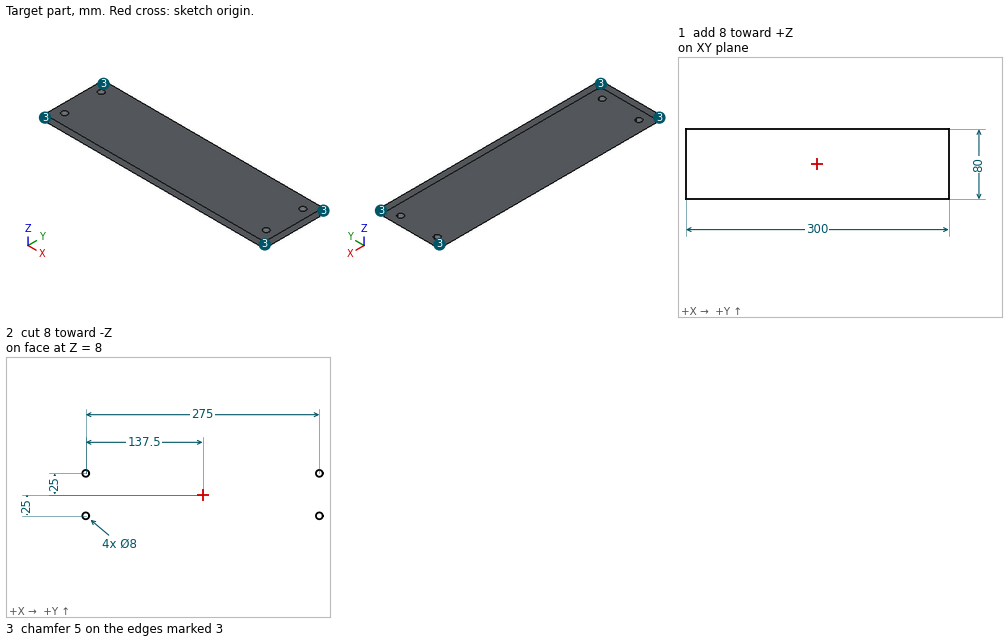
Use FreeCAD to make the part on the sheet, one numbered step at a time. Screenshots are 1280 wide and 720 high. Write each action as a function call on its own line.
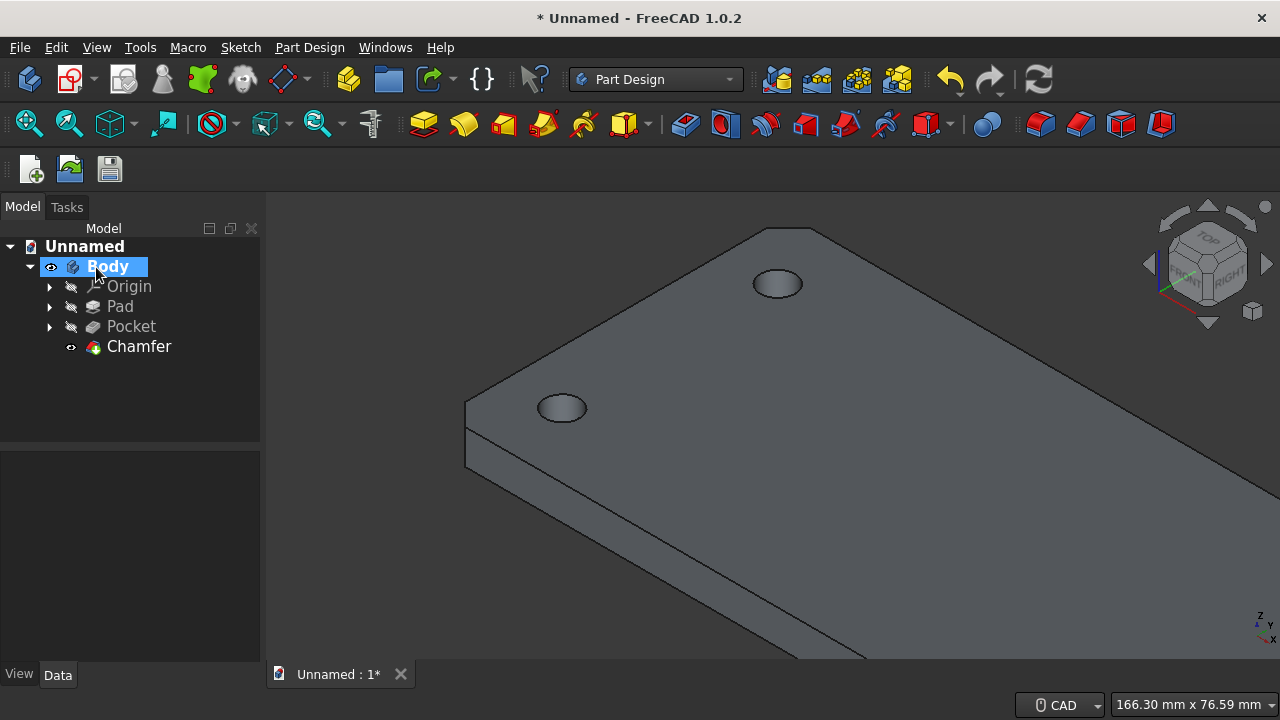
click(30, 124)